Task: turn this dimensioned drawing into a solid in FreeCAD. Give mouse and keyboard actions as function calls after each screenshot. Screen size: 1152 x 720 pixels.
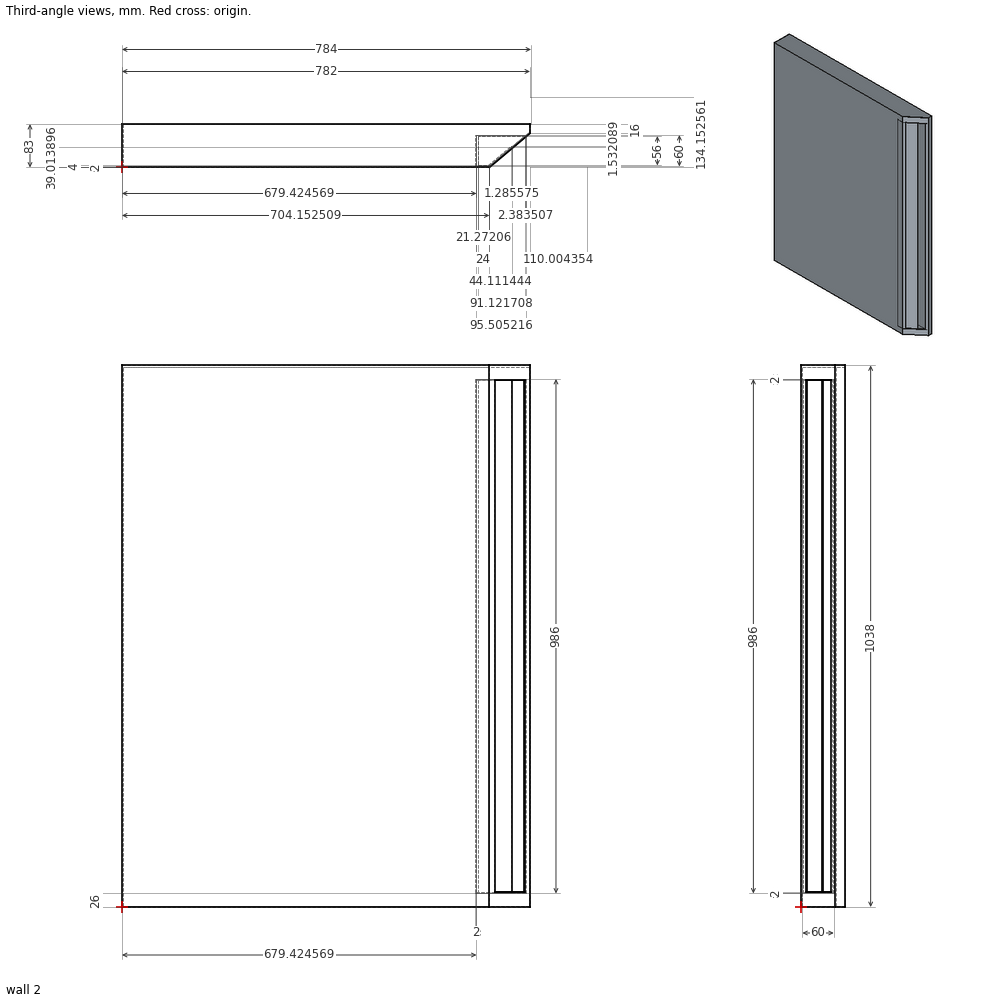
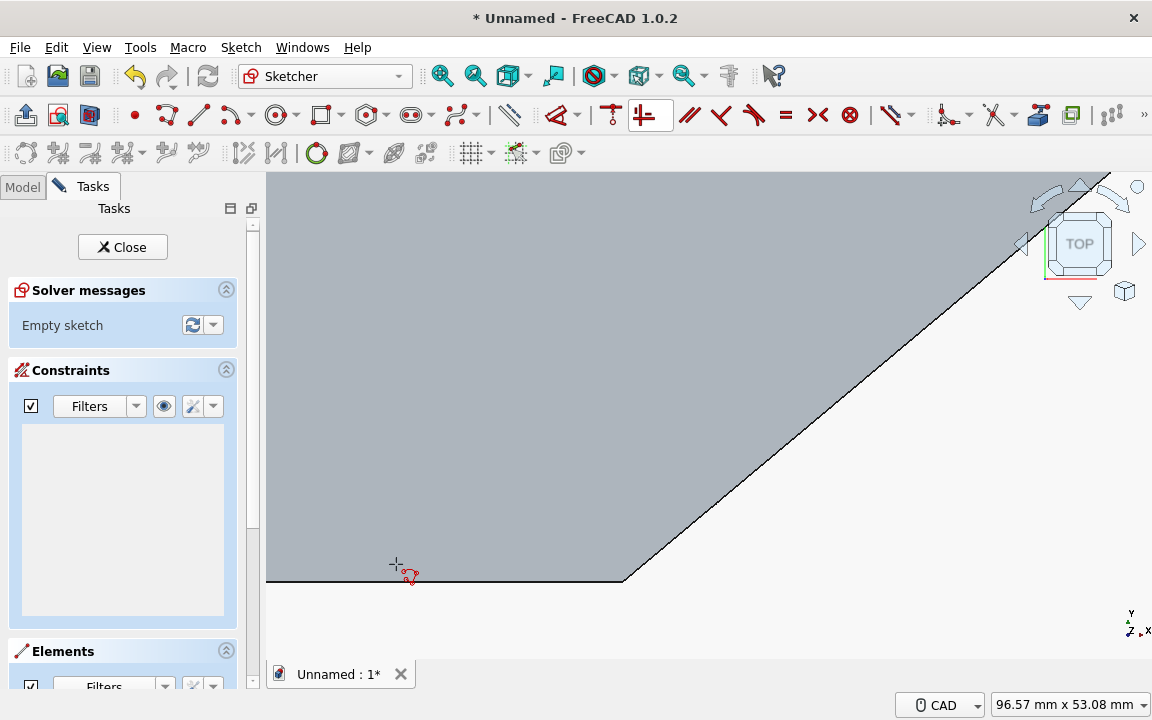
click(395, 564)
click(615, 564)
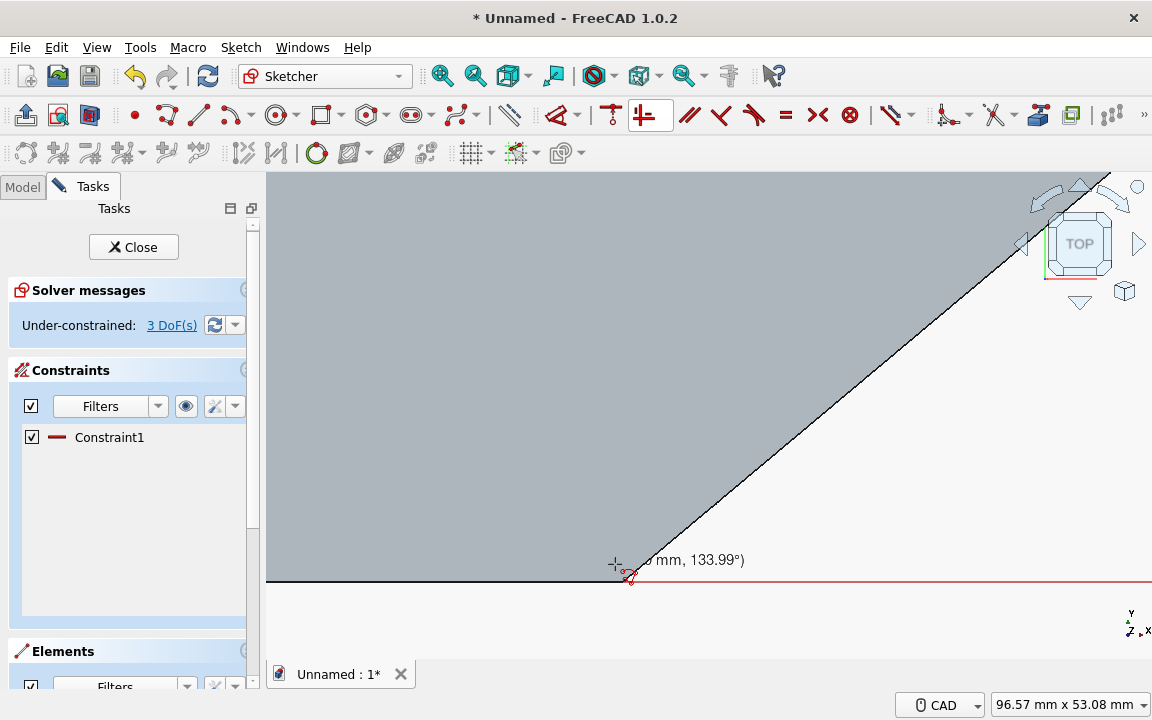
scroll(406, 570, down, 3)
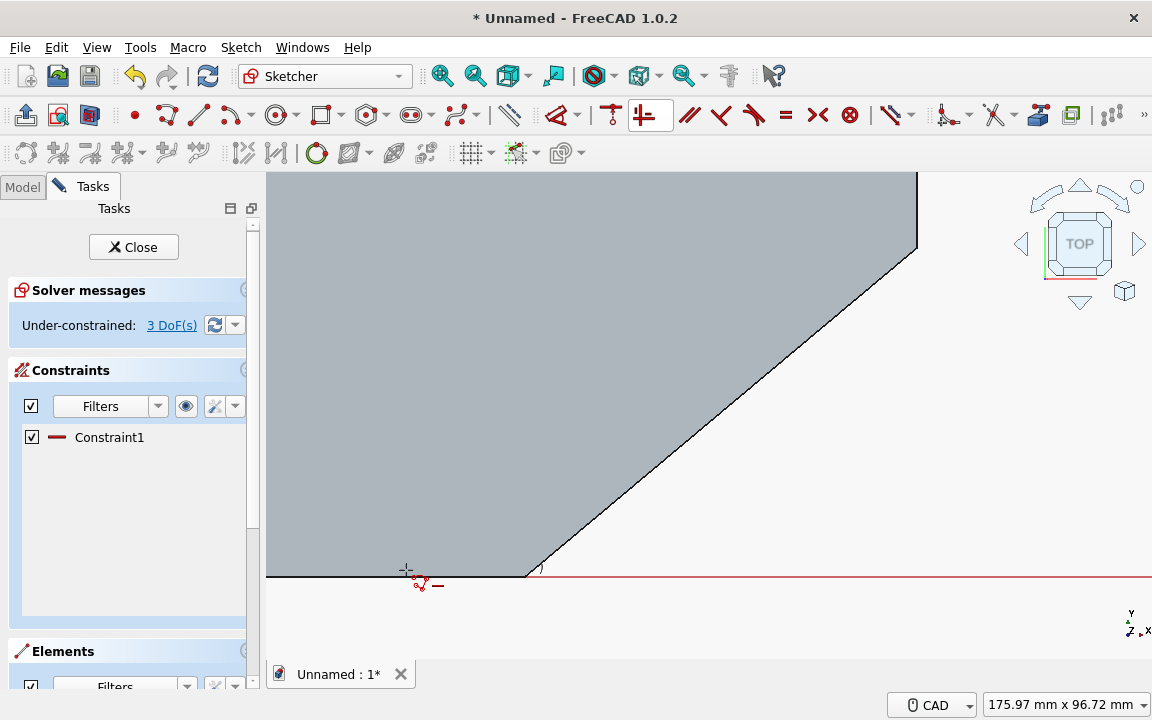
click(743, 381)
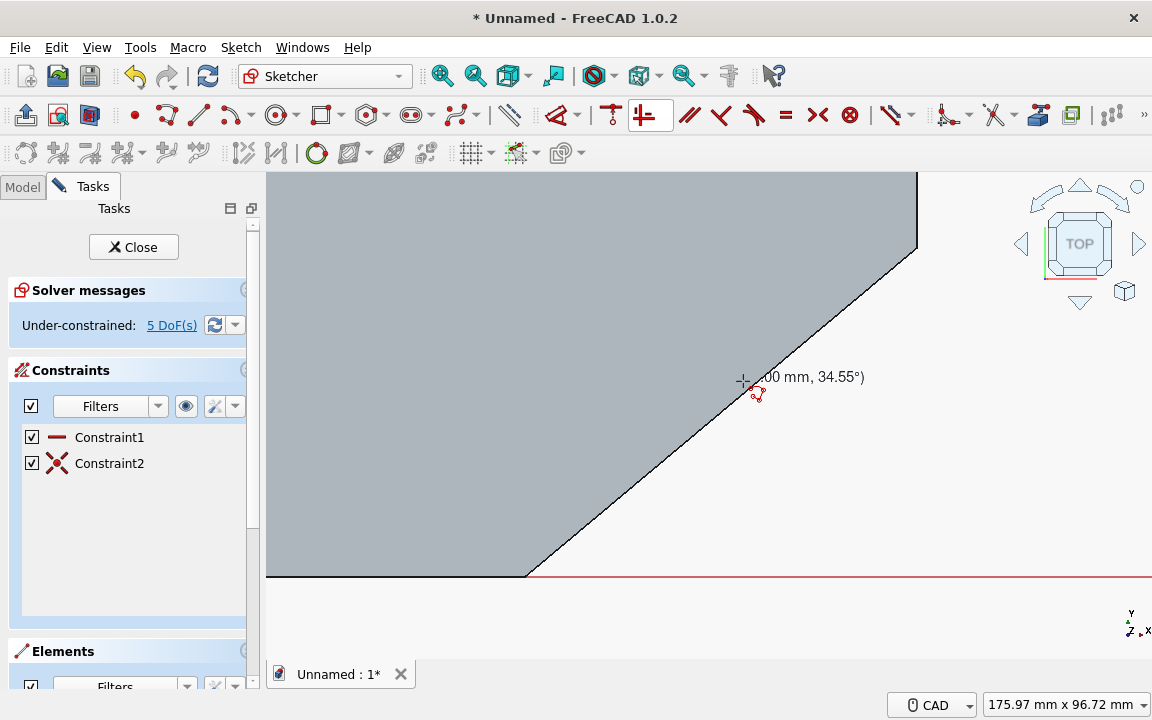
scroll(737, 373, up, 3)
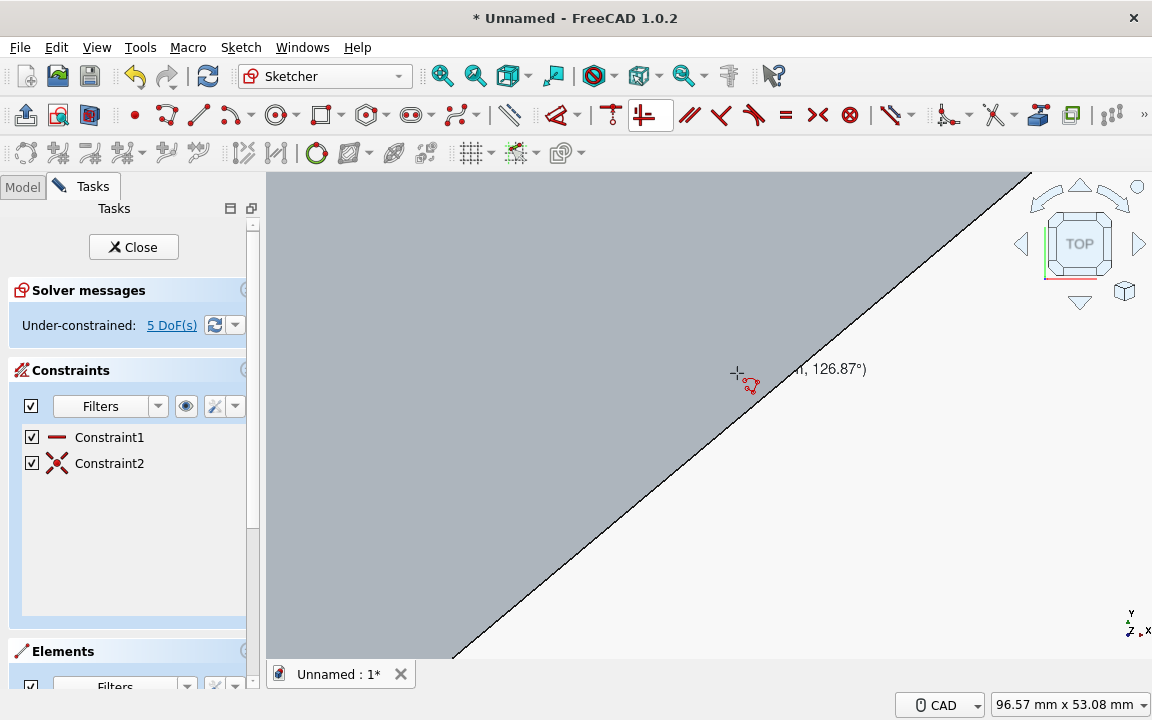
click(736, 373)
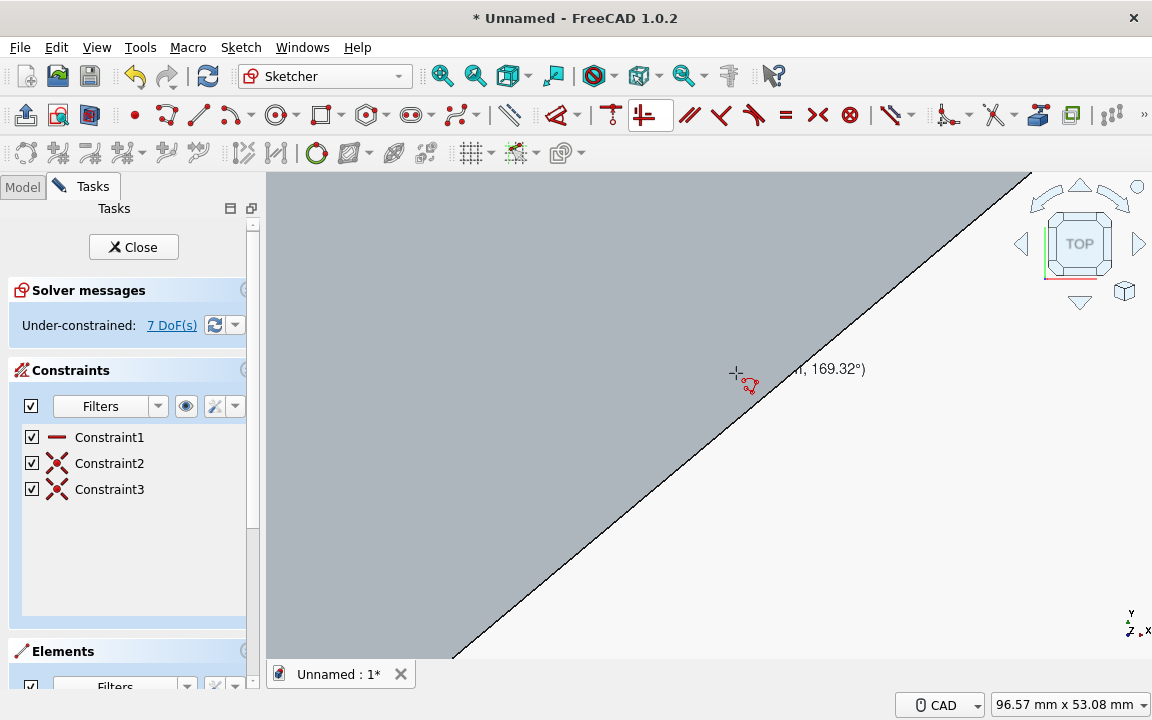
scroll(737, 372, down, 3)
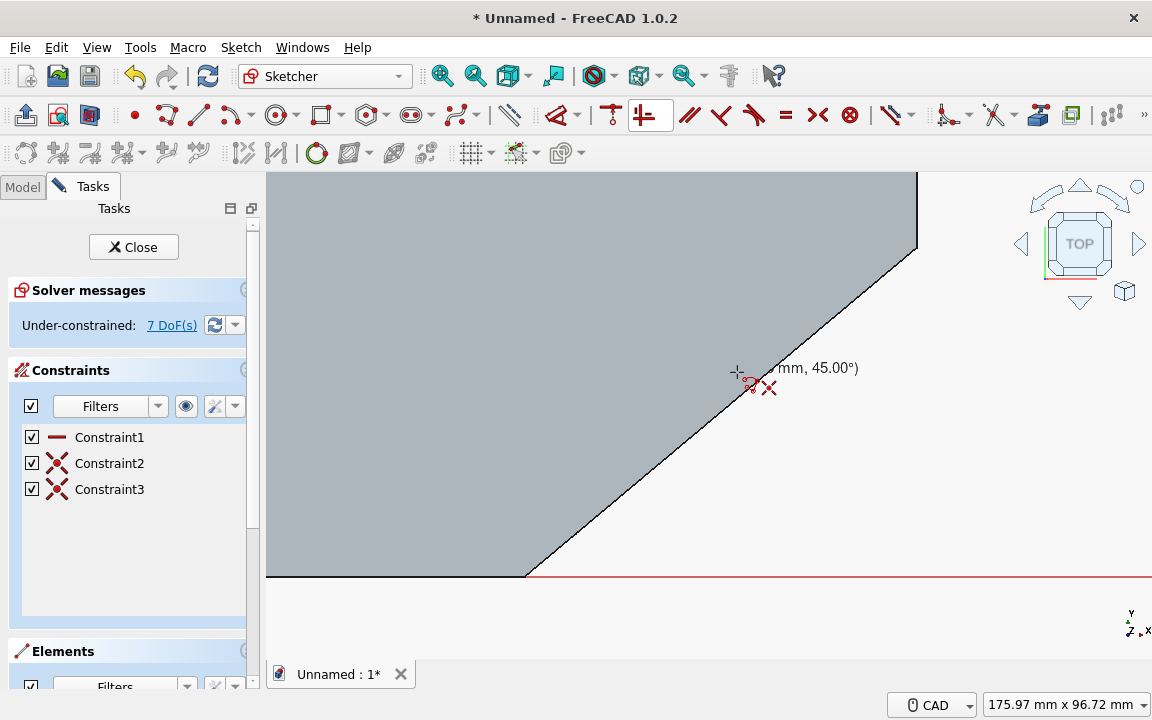
scroll(517, 557, up, 3)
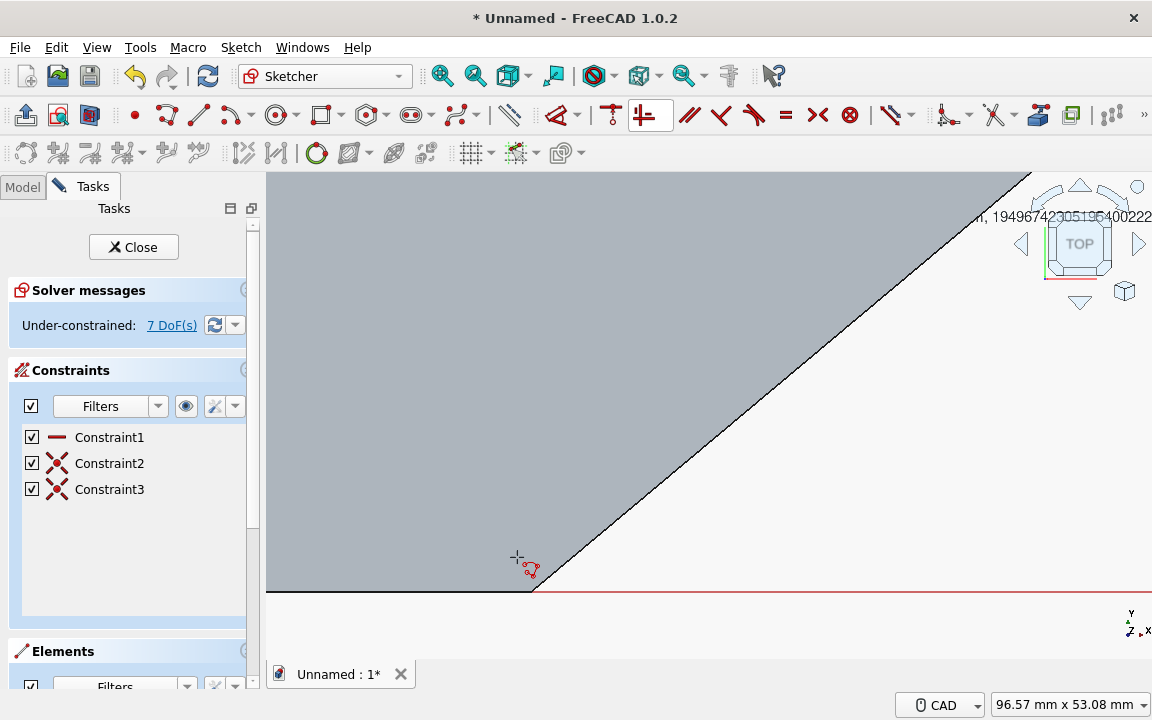
click(517, 556)
click(322, 556)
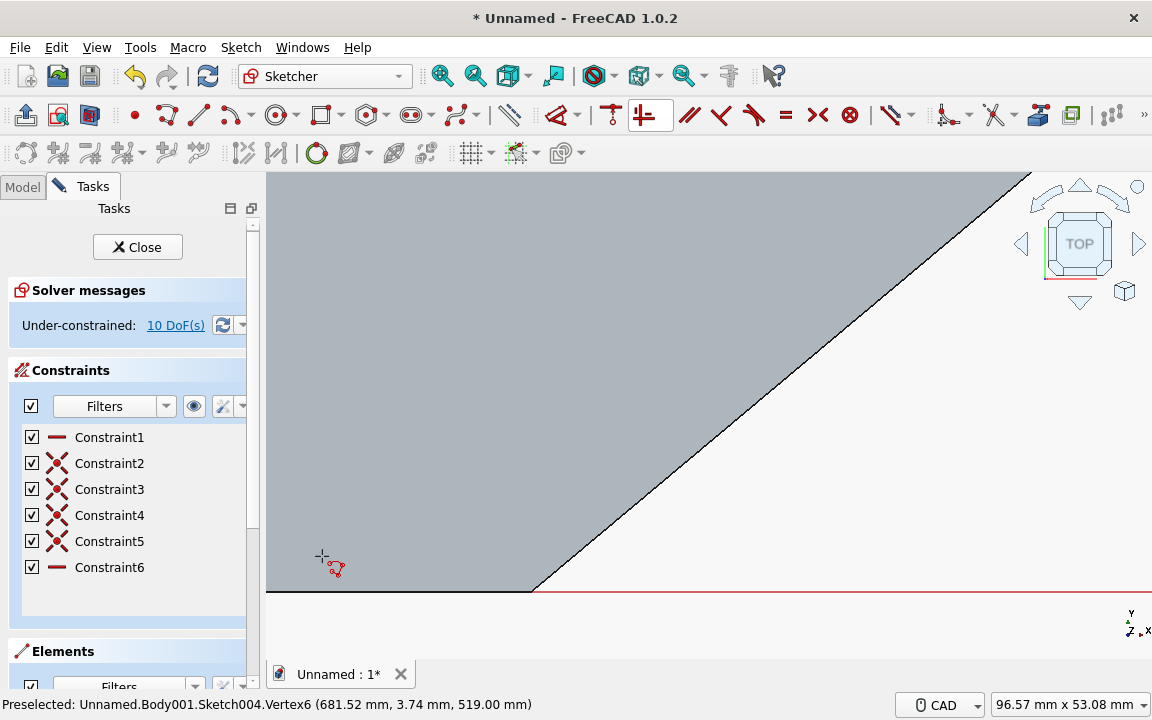
scroll(517, 557, down, 3)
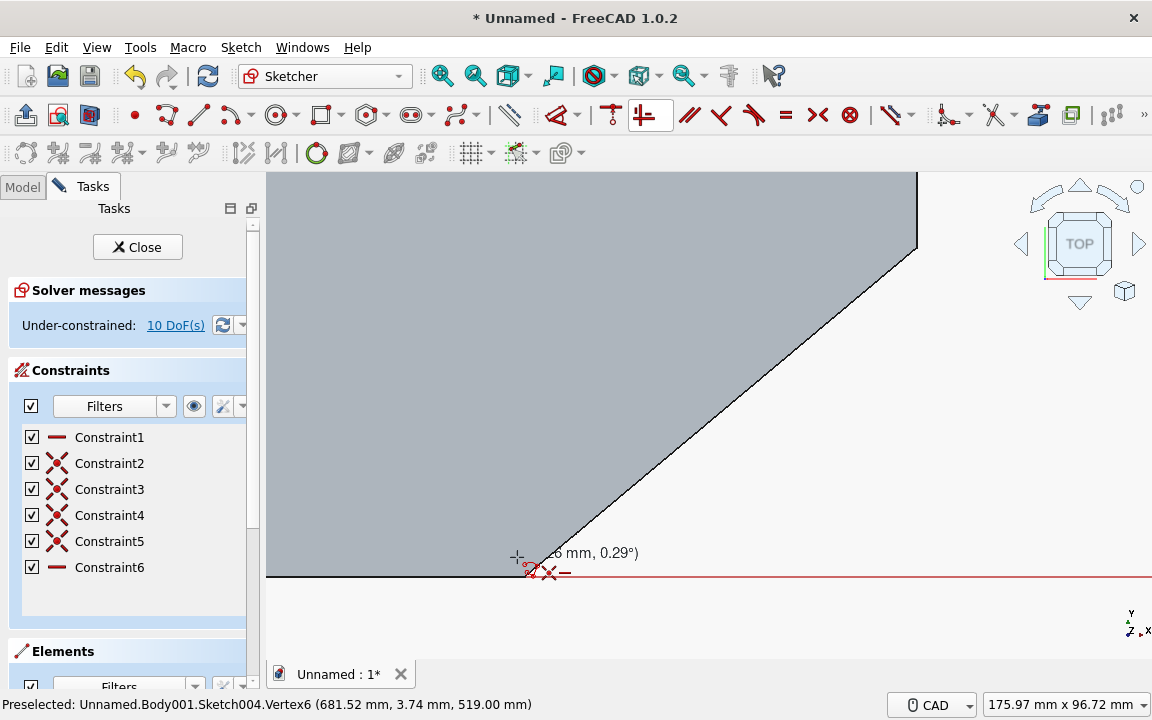
click(410, 275)
click(869, 275)
click(881, 265)
click(400, 265)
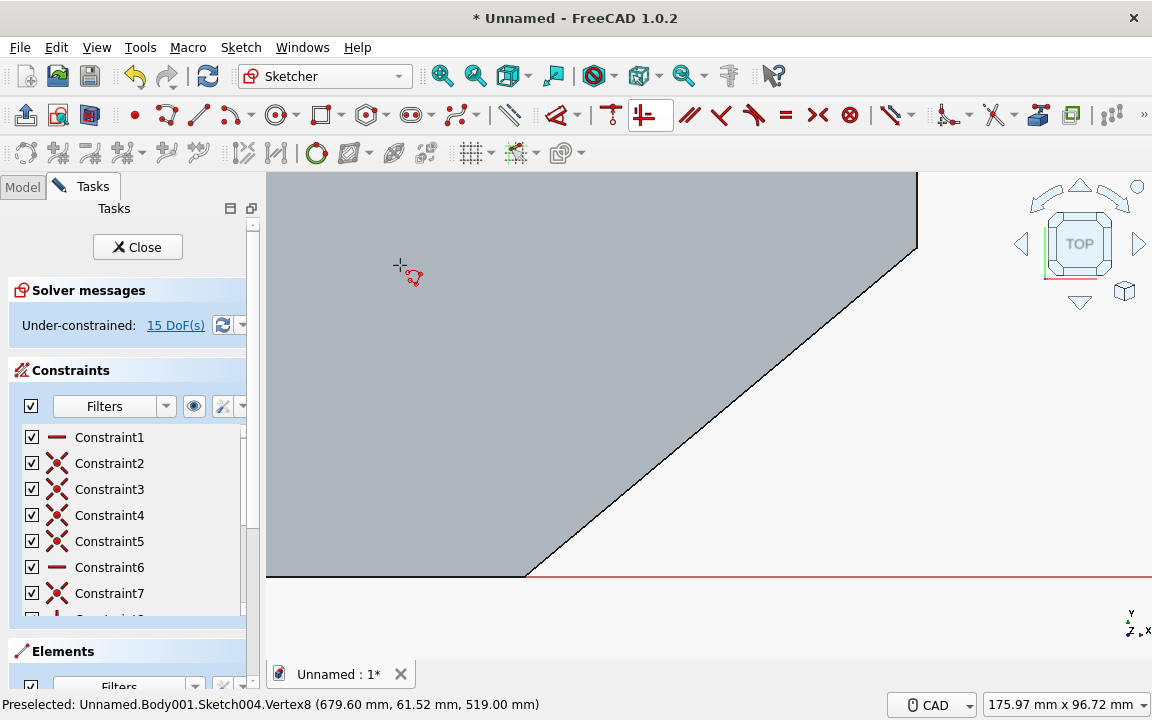
scroll(400, 567, up, 3)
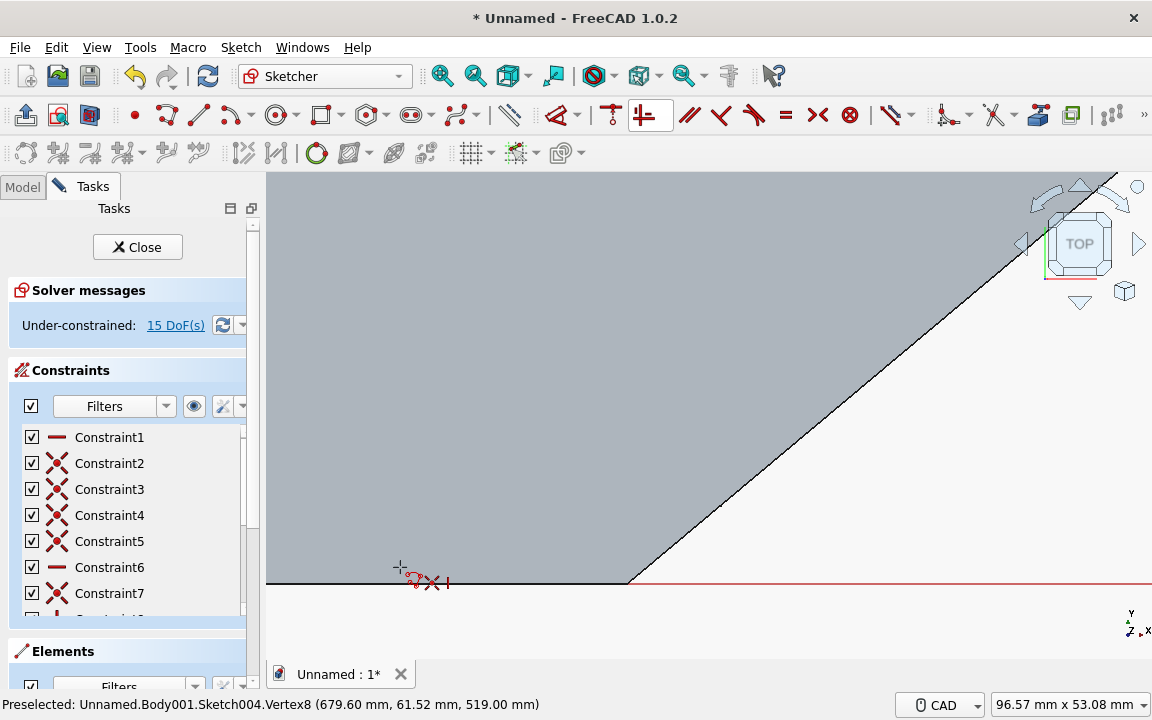
click(400, 567)
key(Escape)
key(Escape)